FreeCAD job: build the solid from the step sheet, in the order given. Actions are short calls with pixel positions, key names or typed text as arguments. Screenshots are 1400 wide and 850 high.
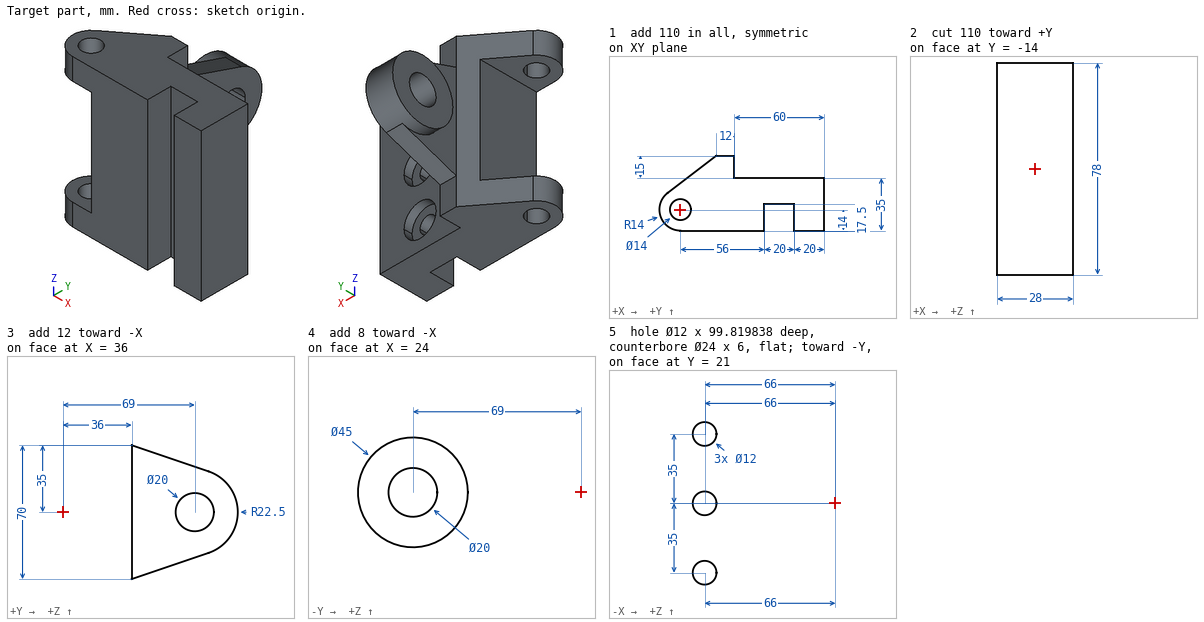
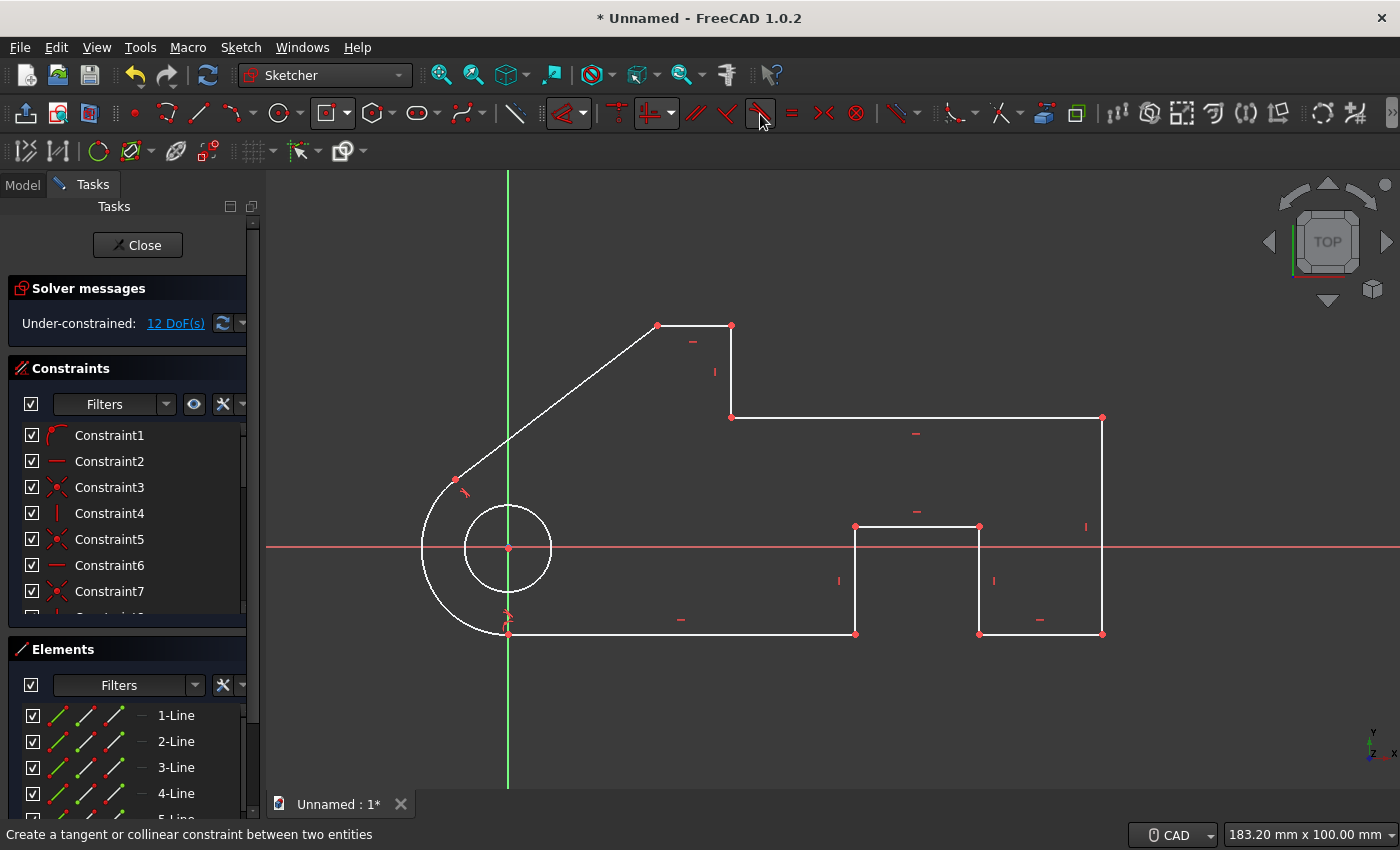
click(508, 549)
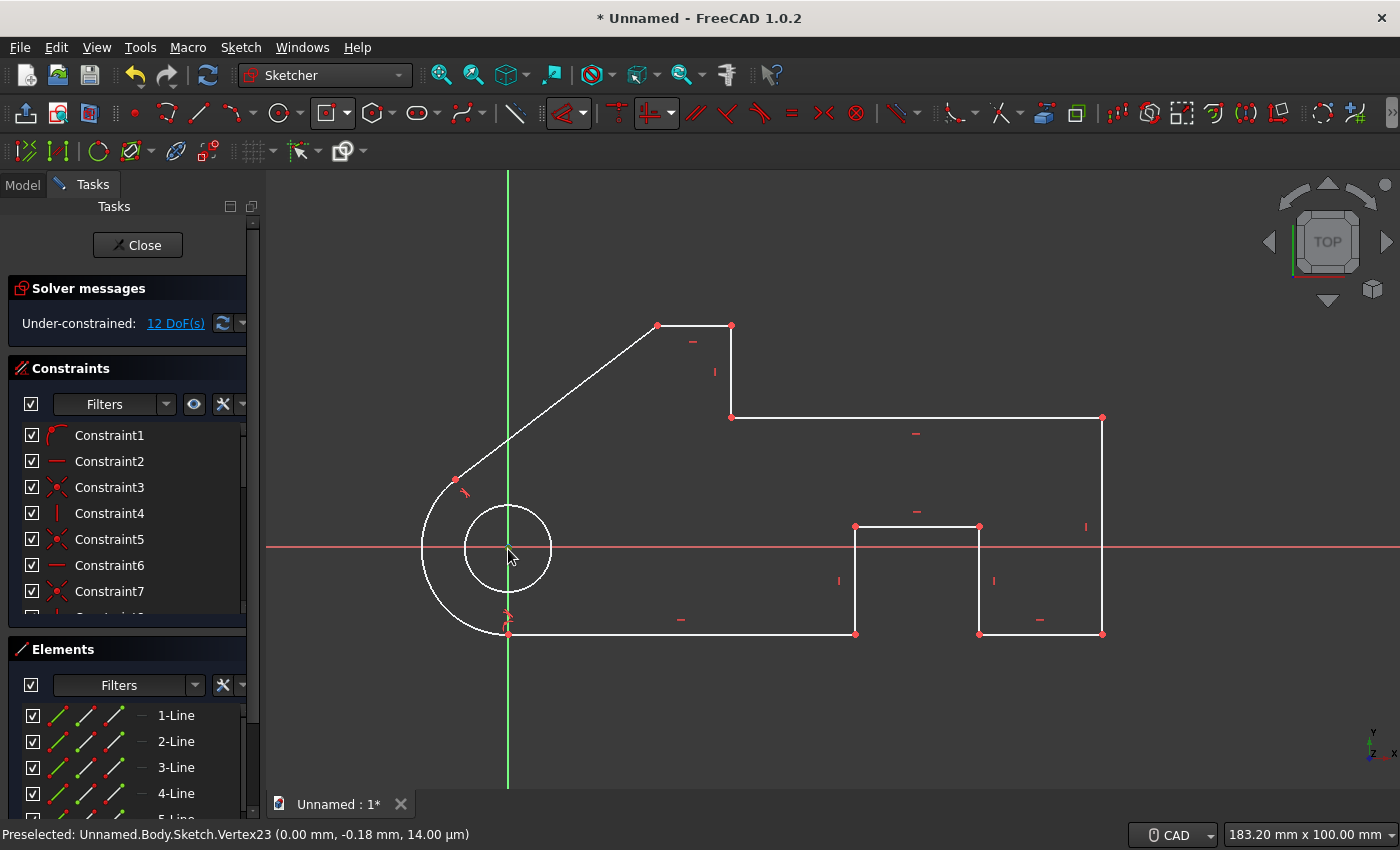
click(361, 547)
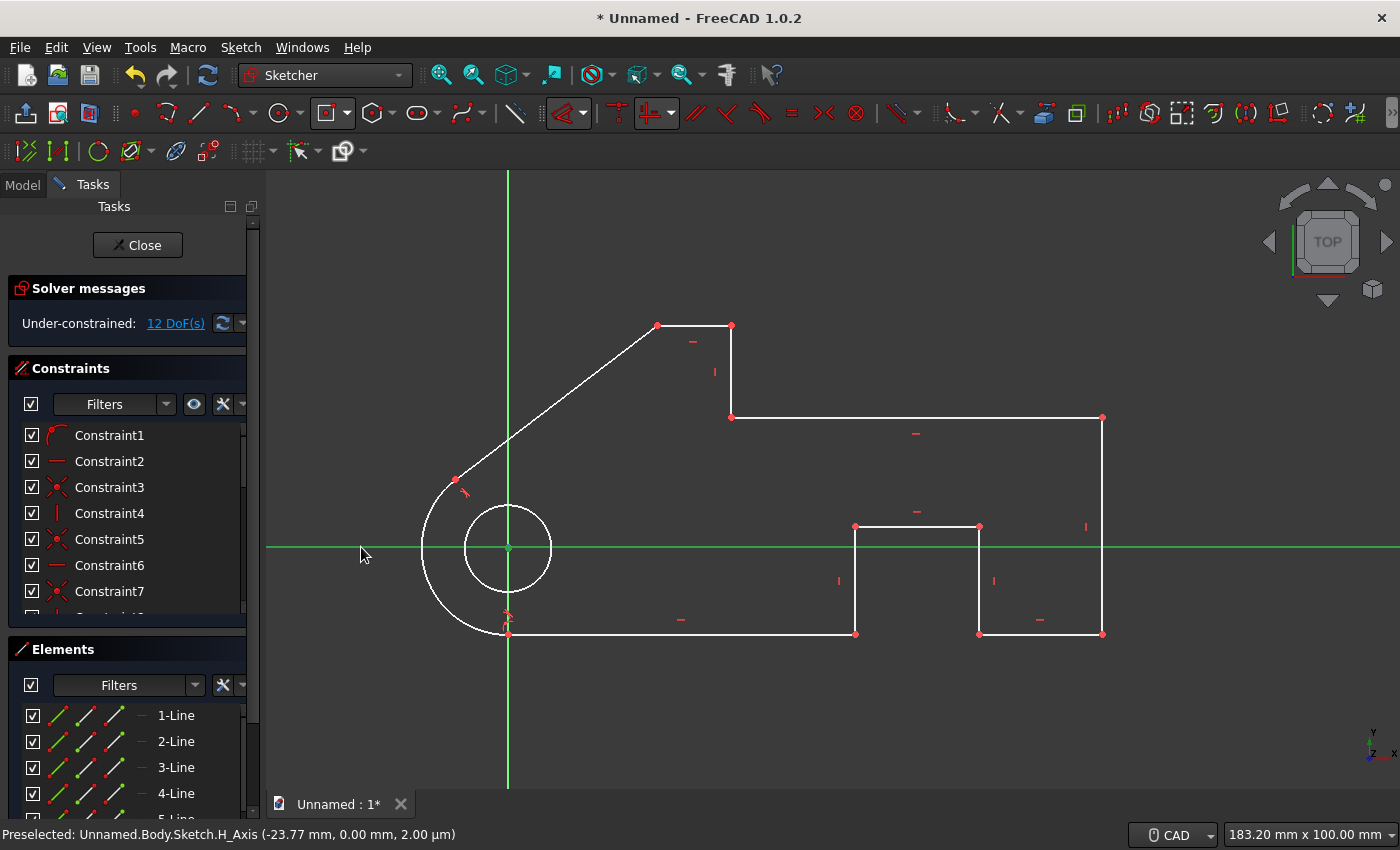
key(c)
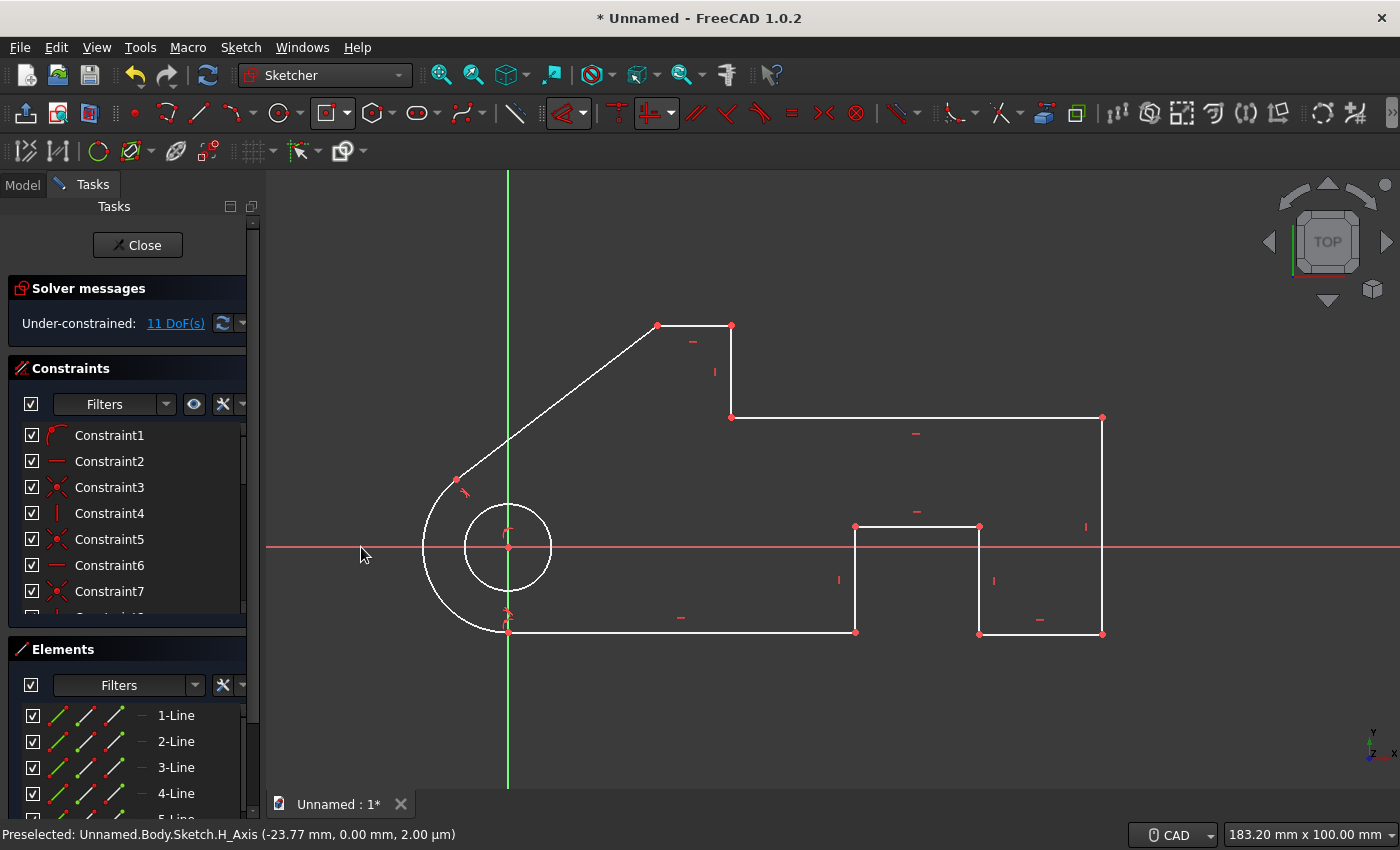
click(562, 114)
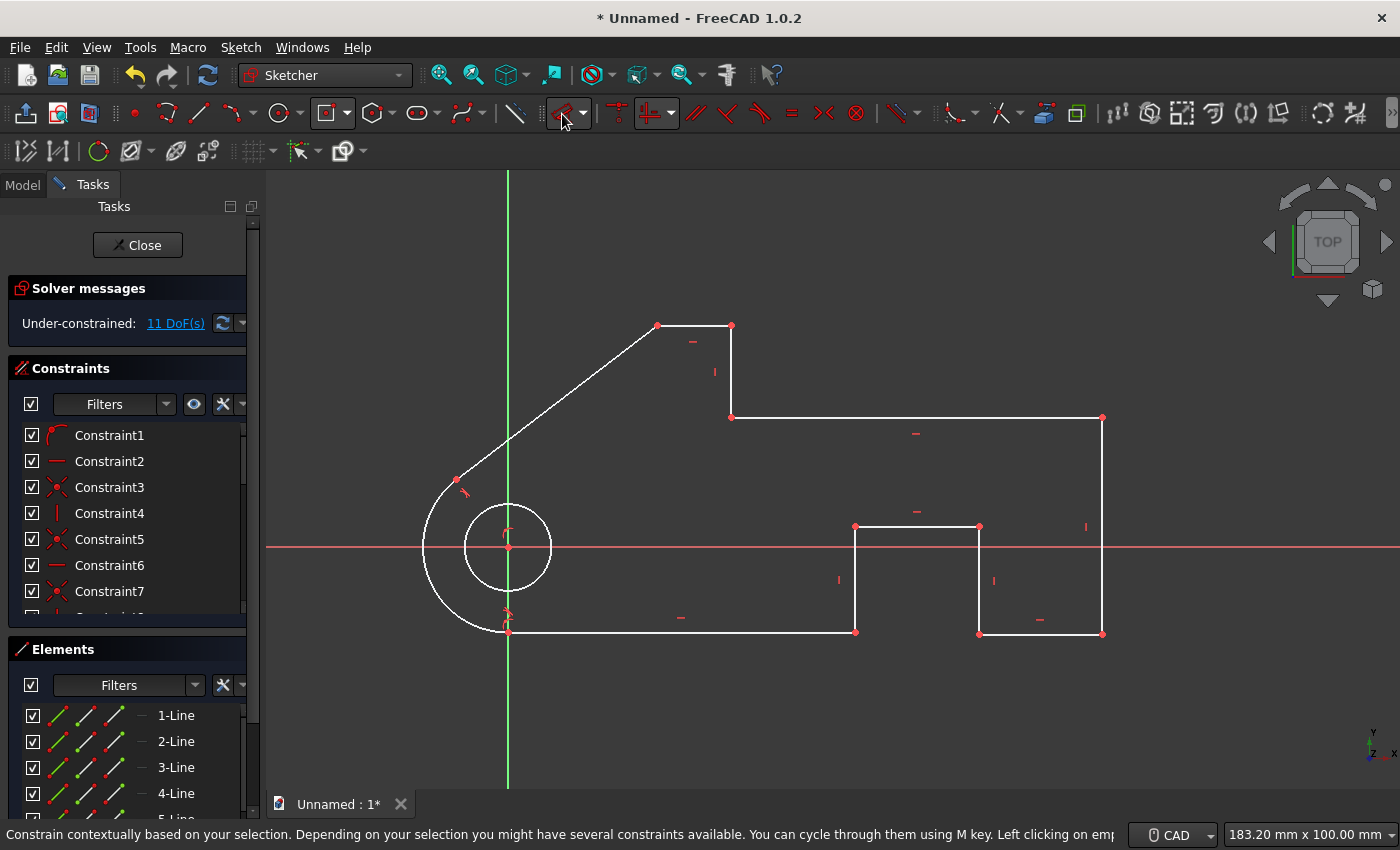
click(424, 533)
click(392, 528)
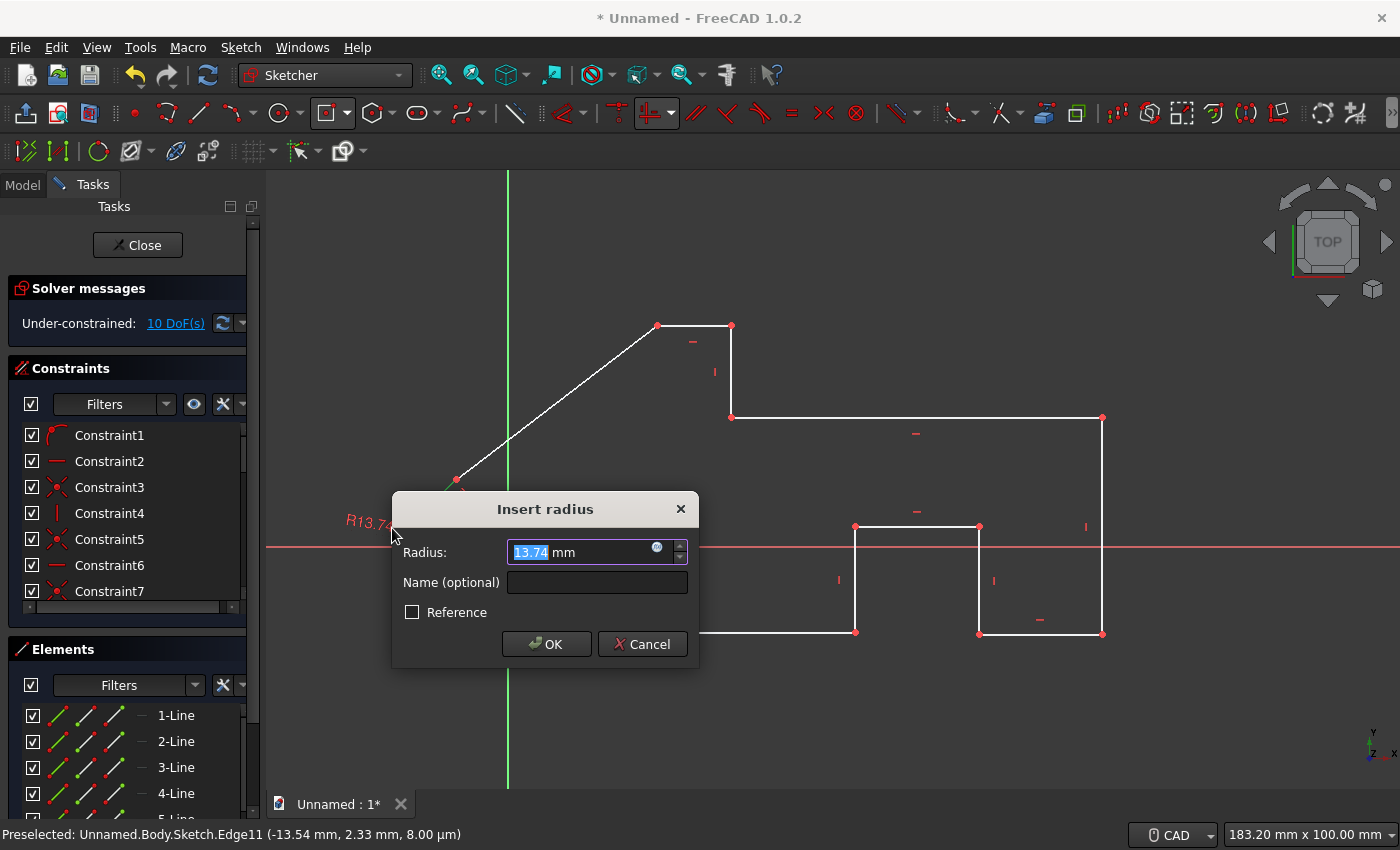
text(14)
key(Return)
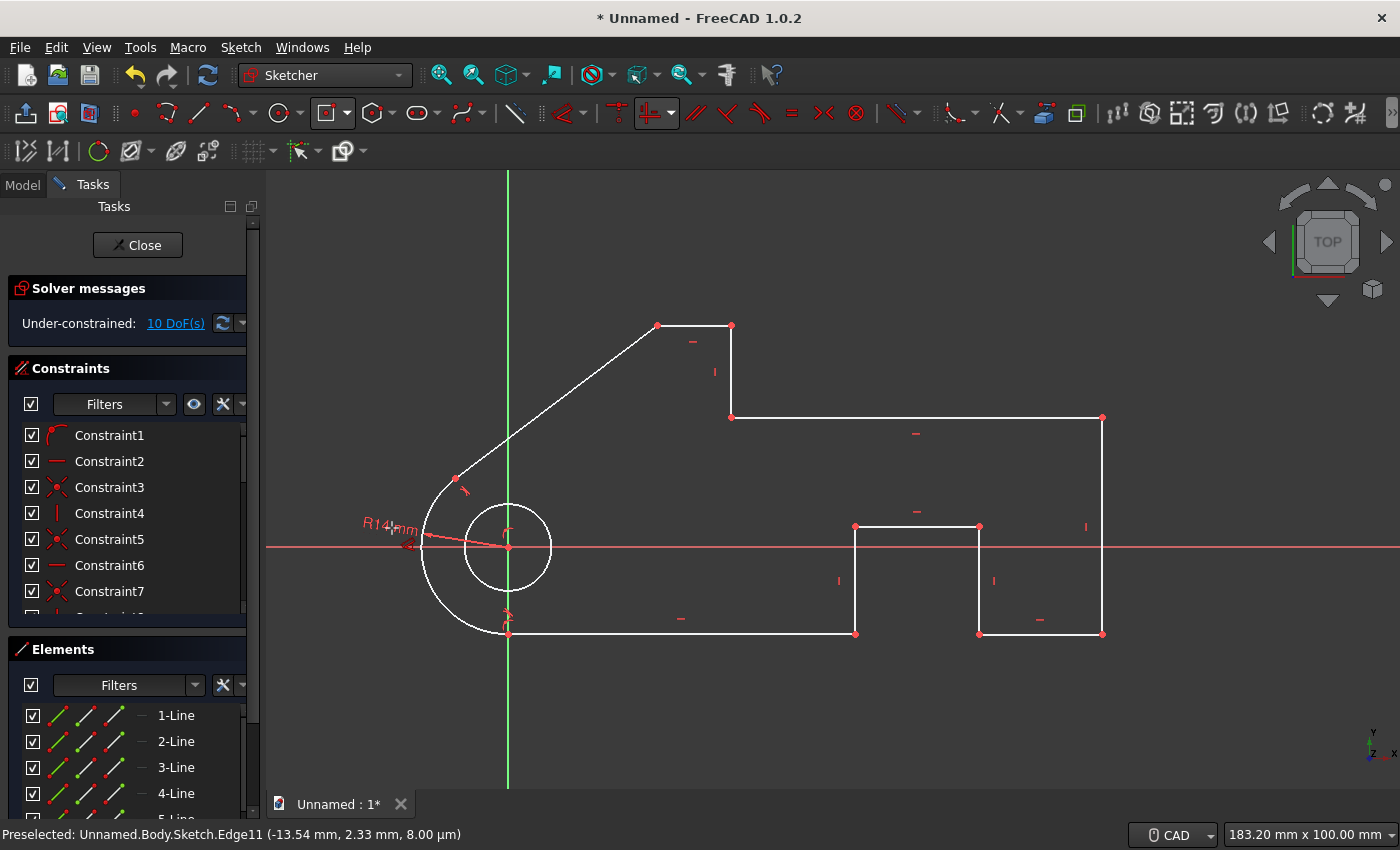
click(539, 517)
click(562, 495)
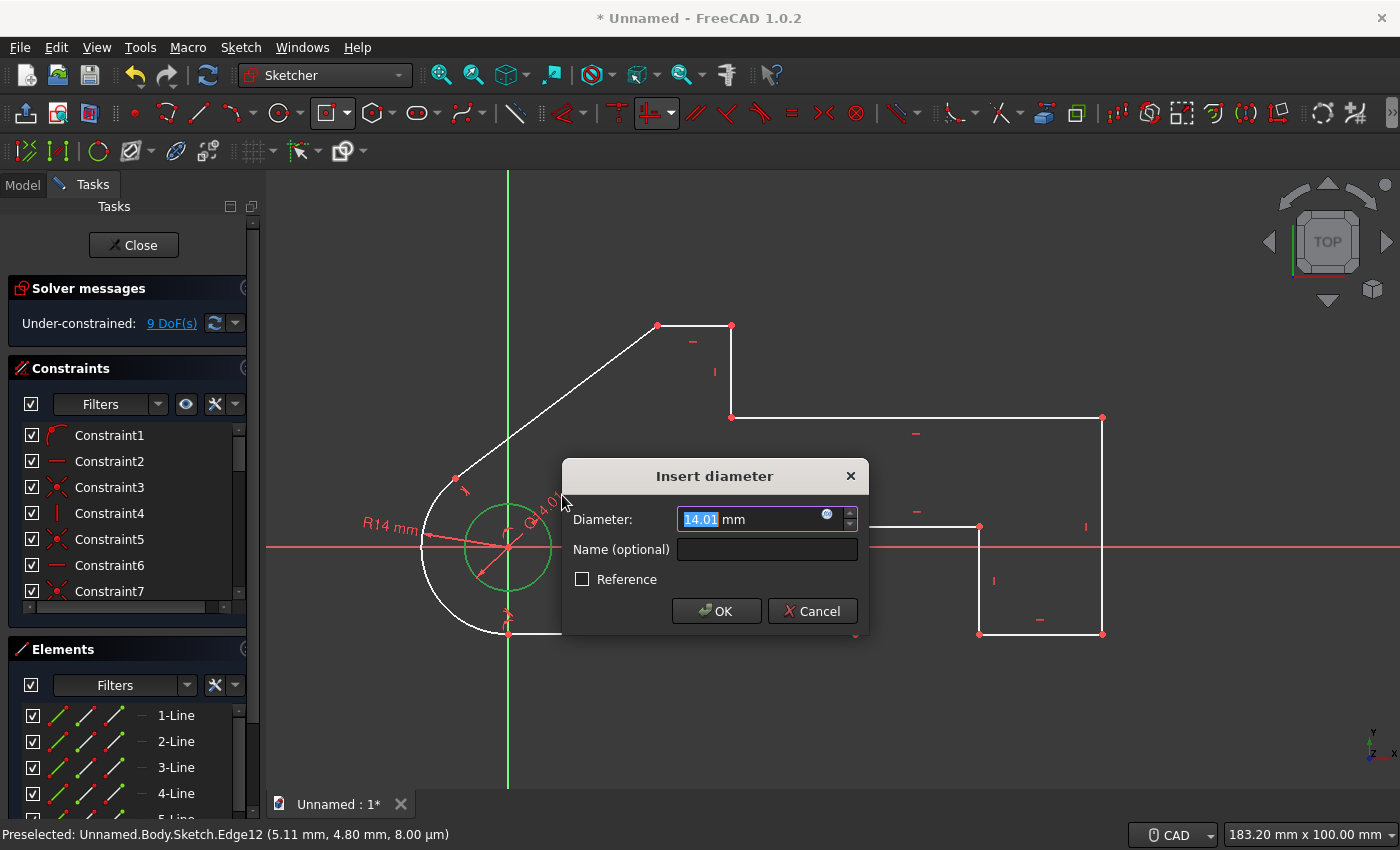
text(14)
key(Return)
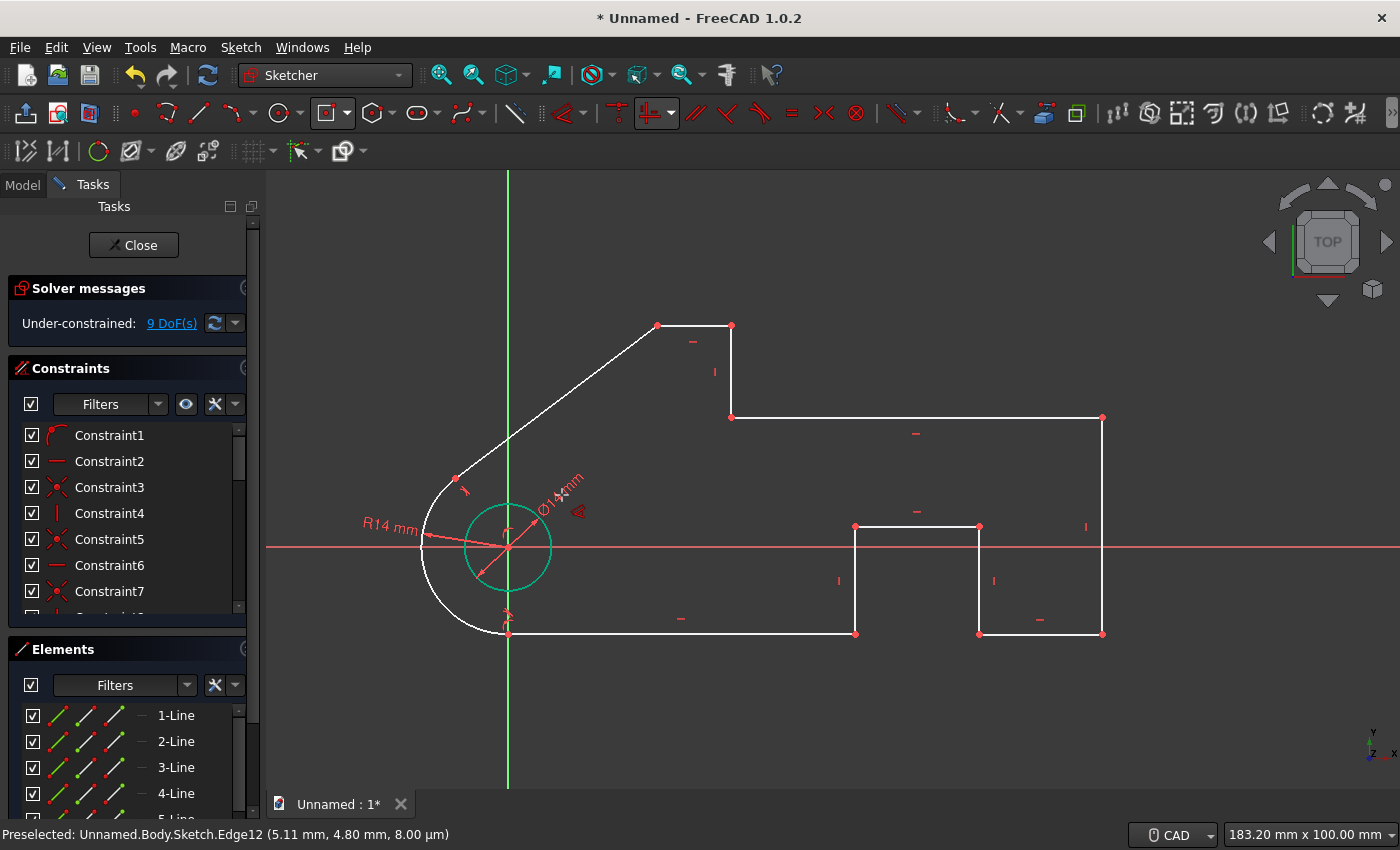
click(612, 634)
click(682, 668)